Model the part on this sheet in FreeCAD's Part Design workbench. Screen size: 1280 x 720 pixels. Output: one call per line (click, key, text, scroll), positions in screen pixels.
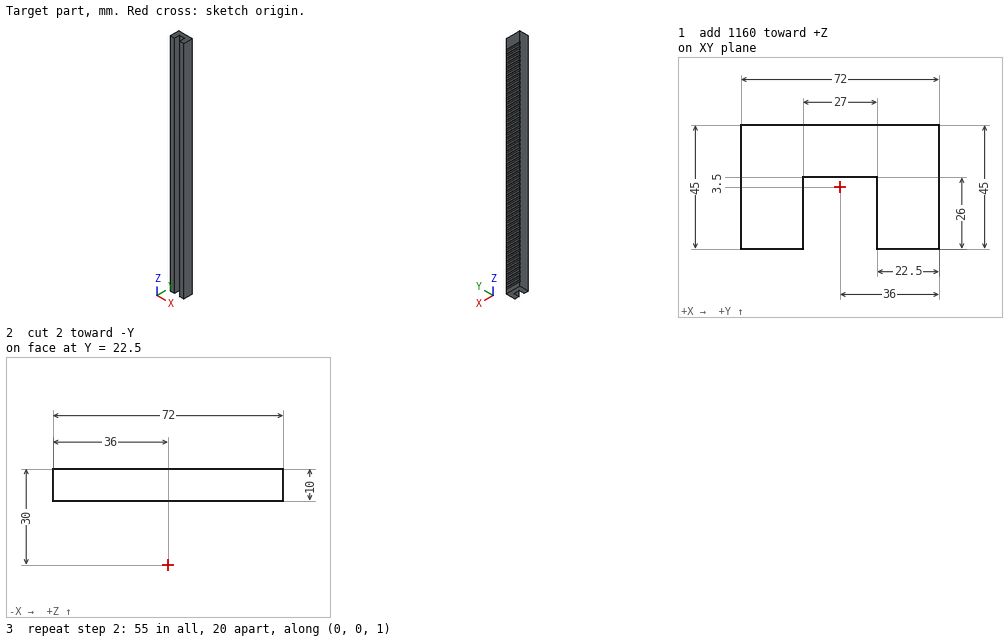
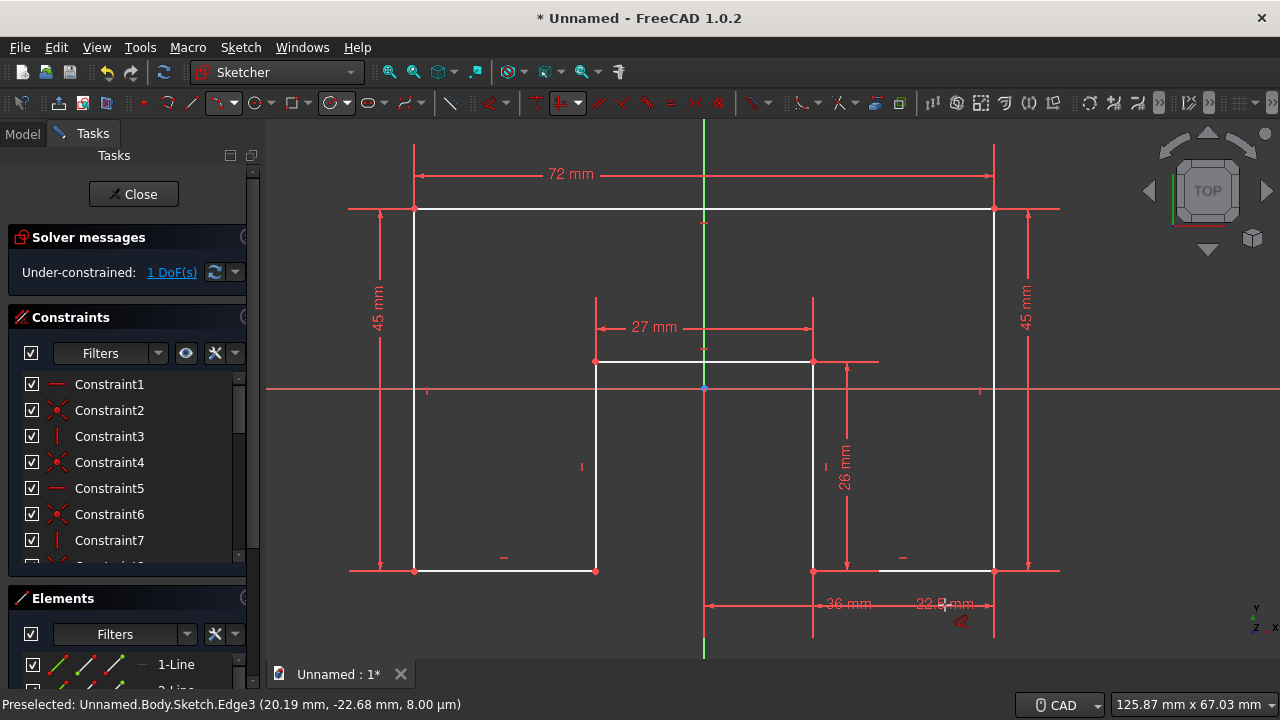
scroll(596, 362, up, 2)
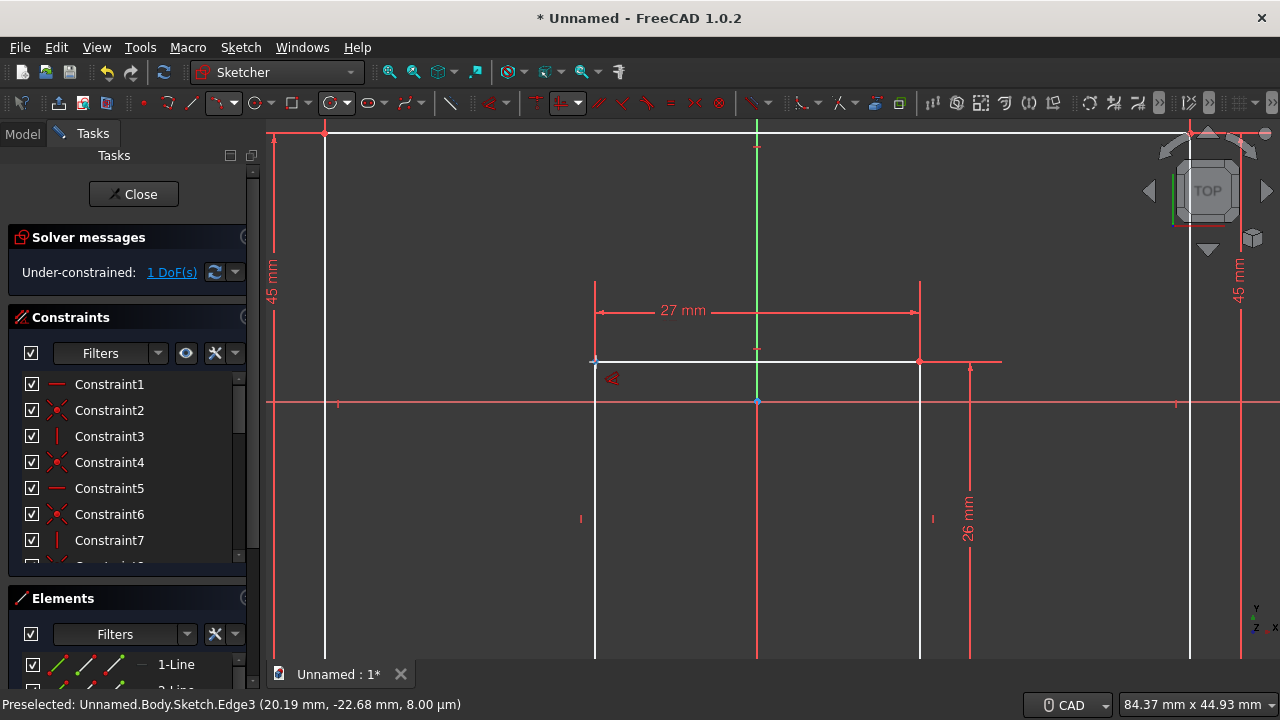
click(595, 362)
click(561, 382)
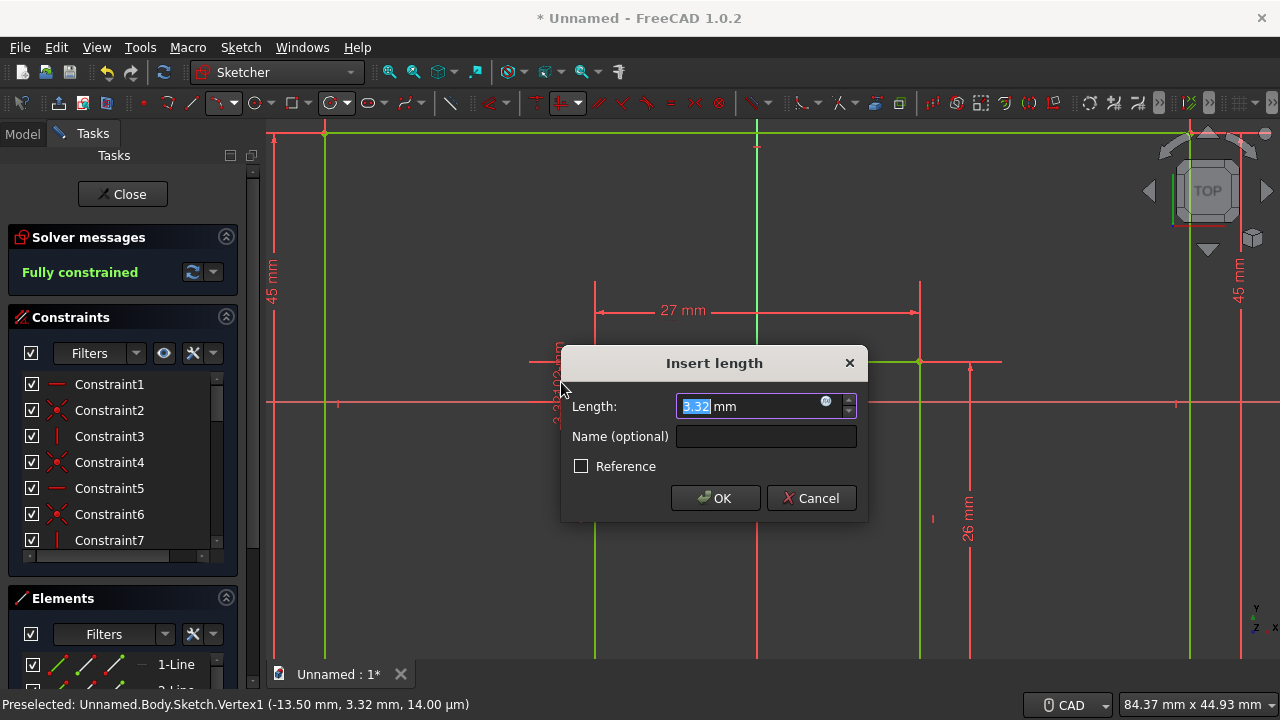
text(3.5)
key(Return)
key(Escape)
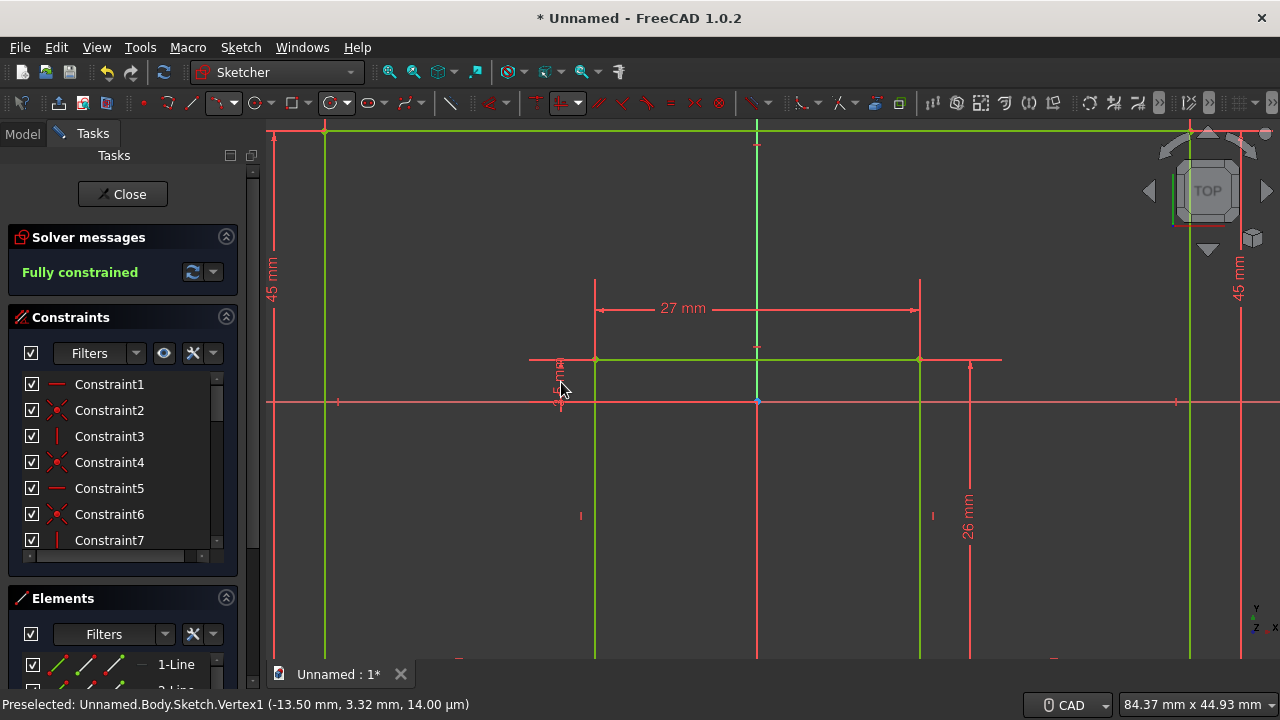
click(123, 194)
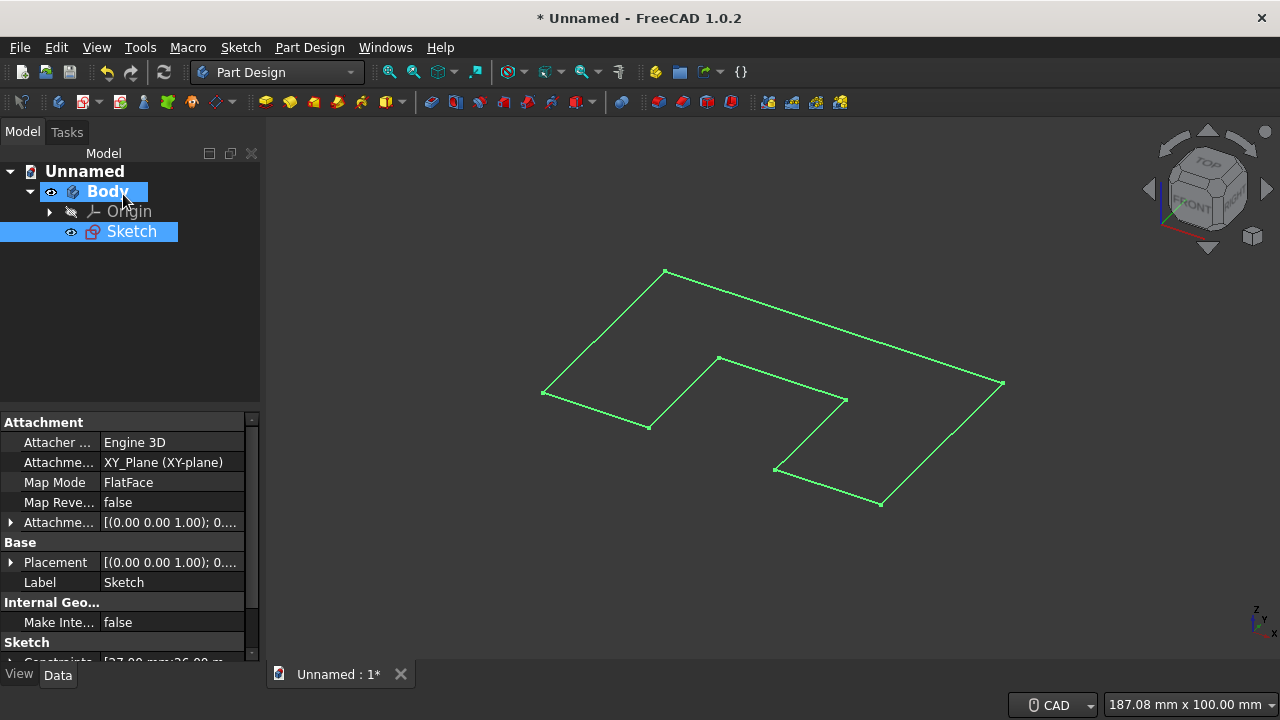
click(266, 102)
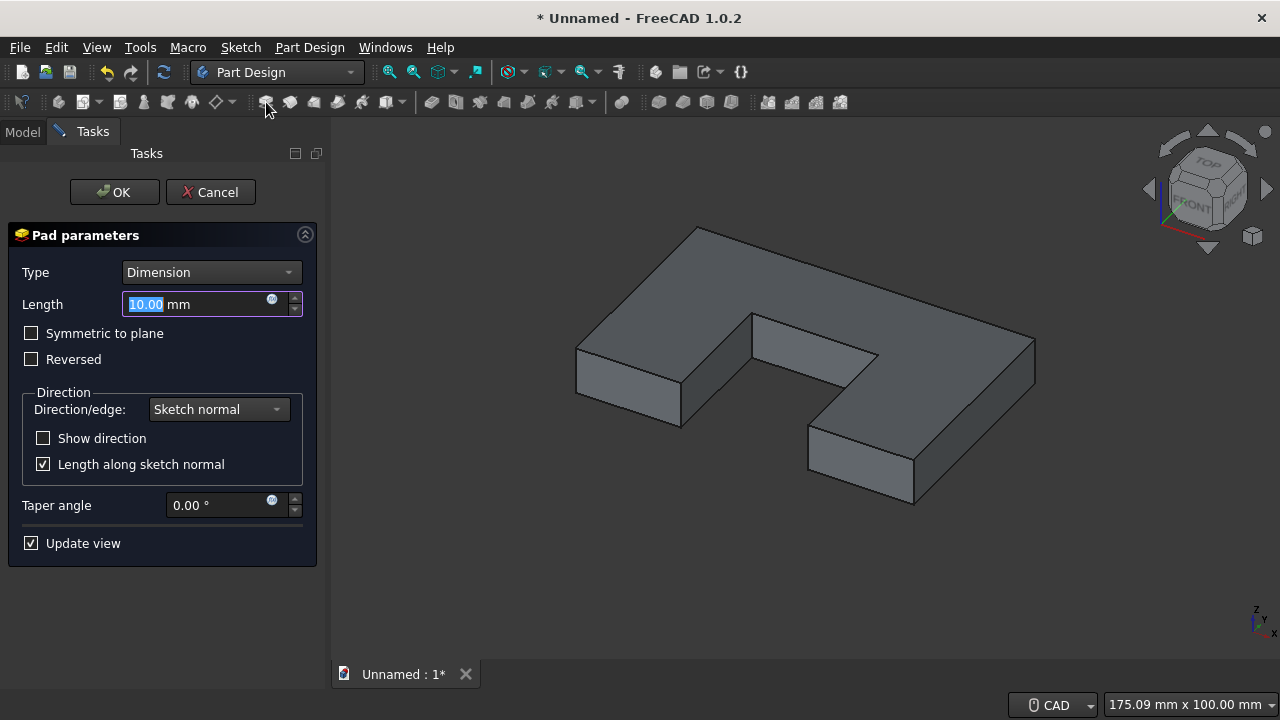
text(1160)
key(Tab)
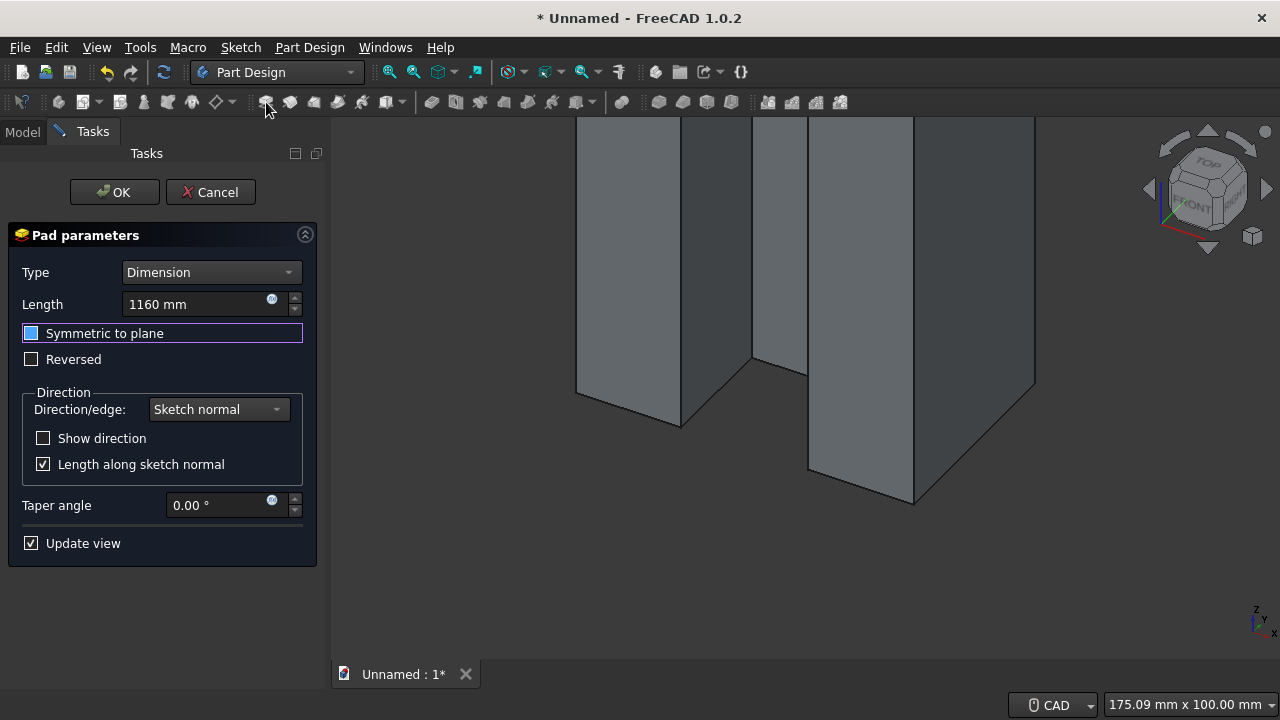
click(115, 192)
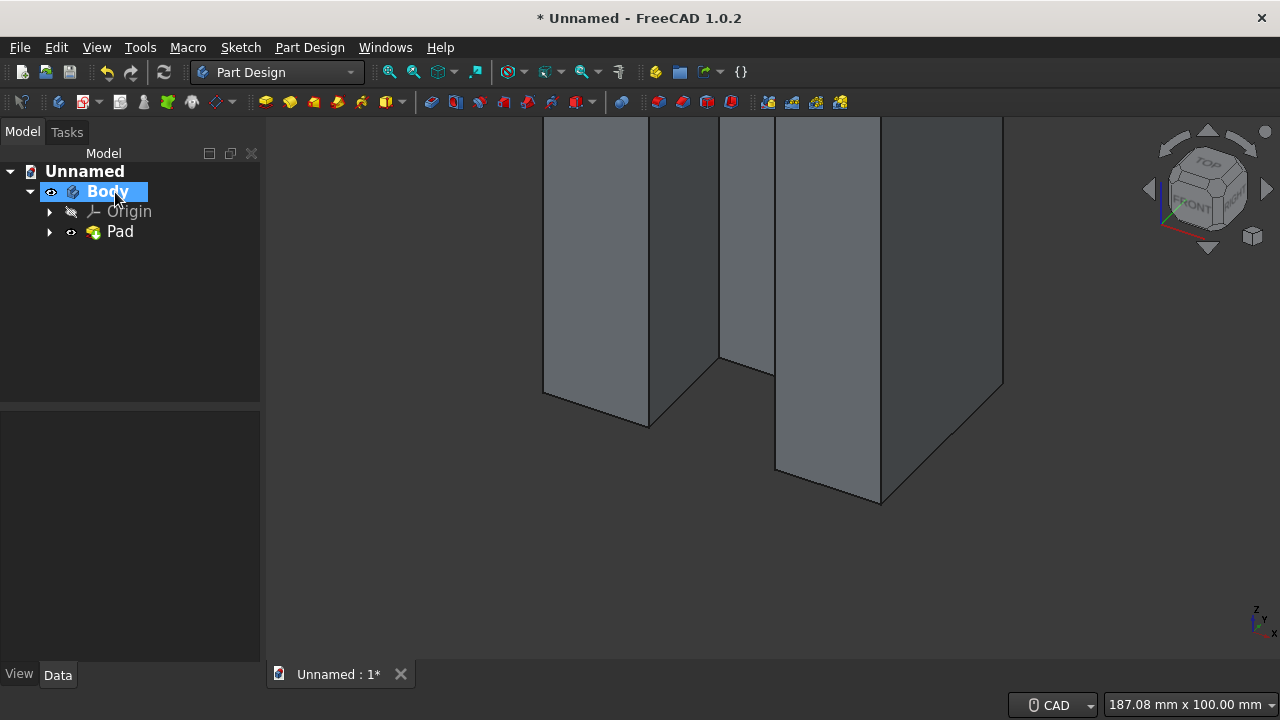
click(390, 72)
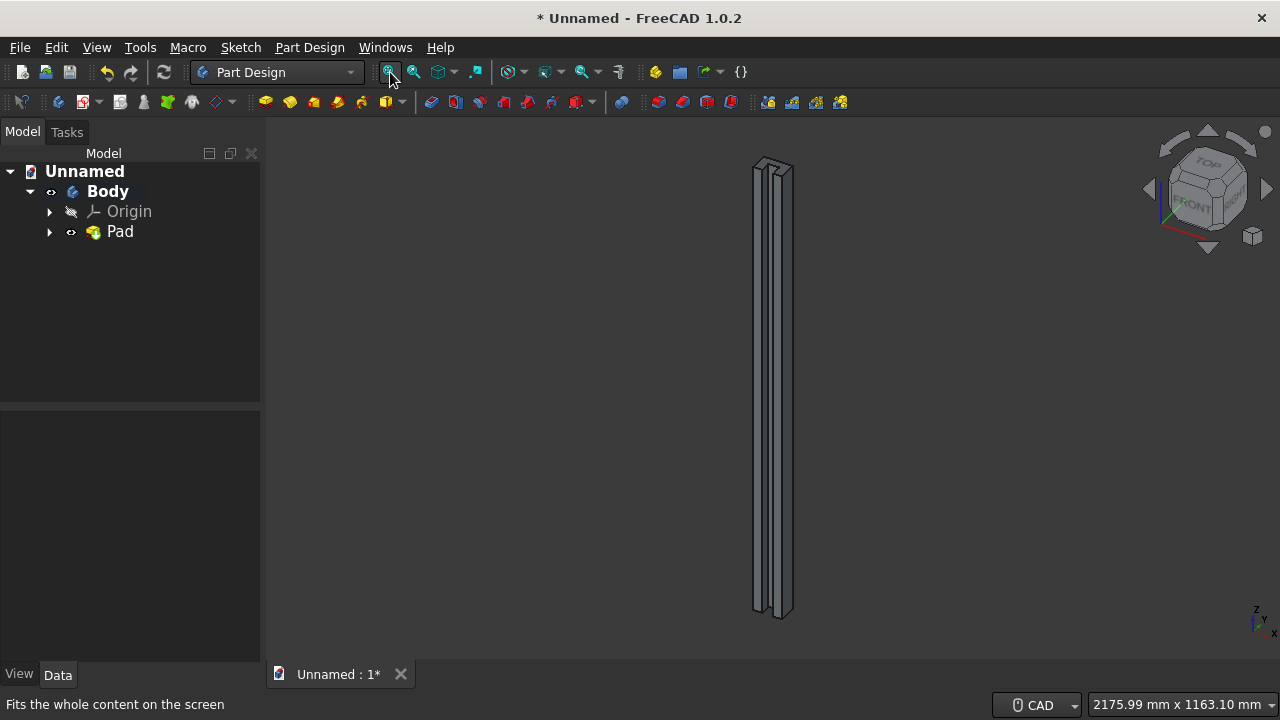
key(4)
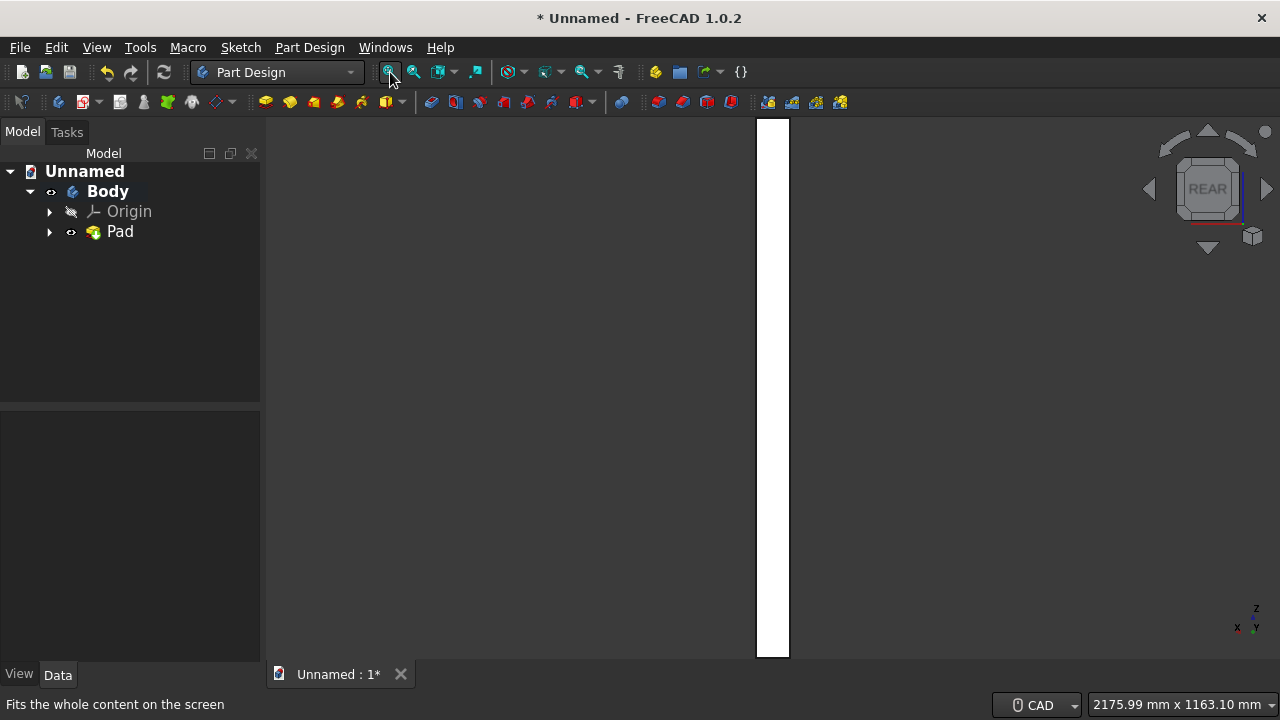
click(773, 155)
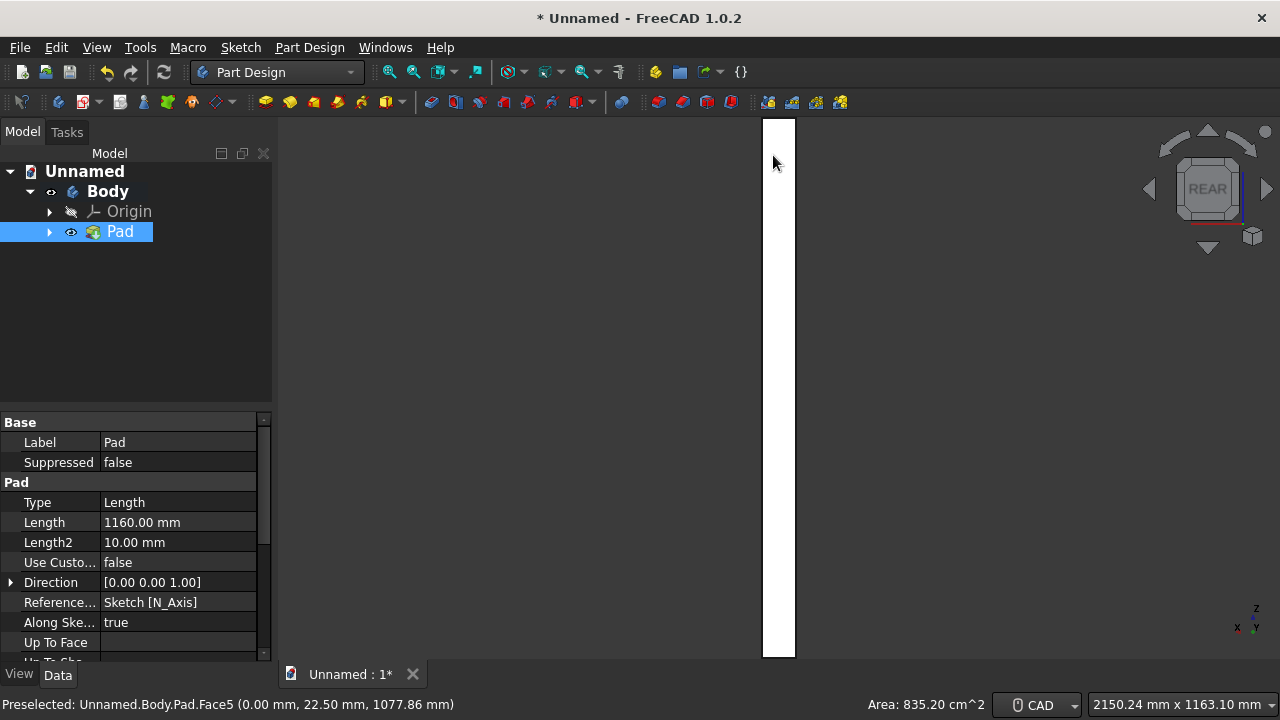
click(84, 102)